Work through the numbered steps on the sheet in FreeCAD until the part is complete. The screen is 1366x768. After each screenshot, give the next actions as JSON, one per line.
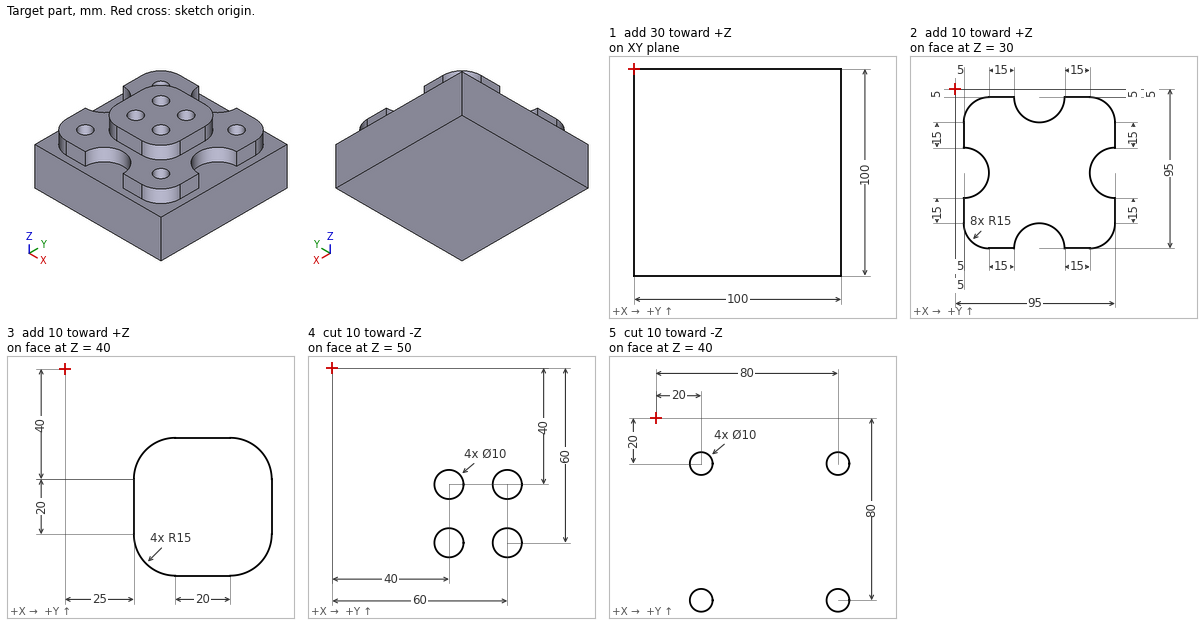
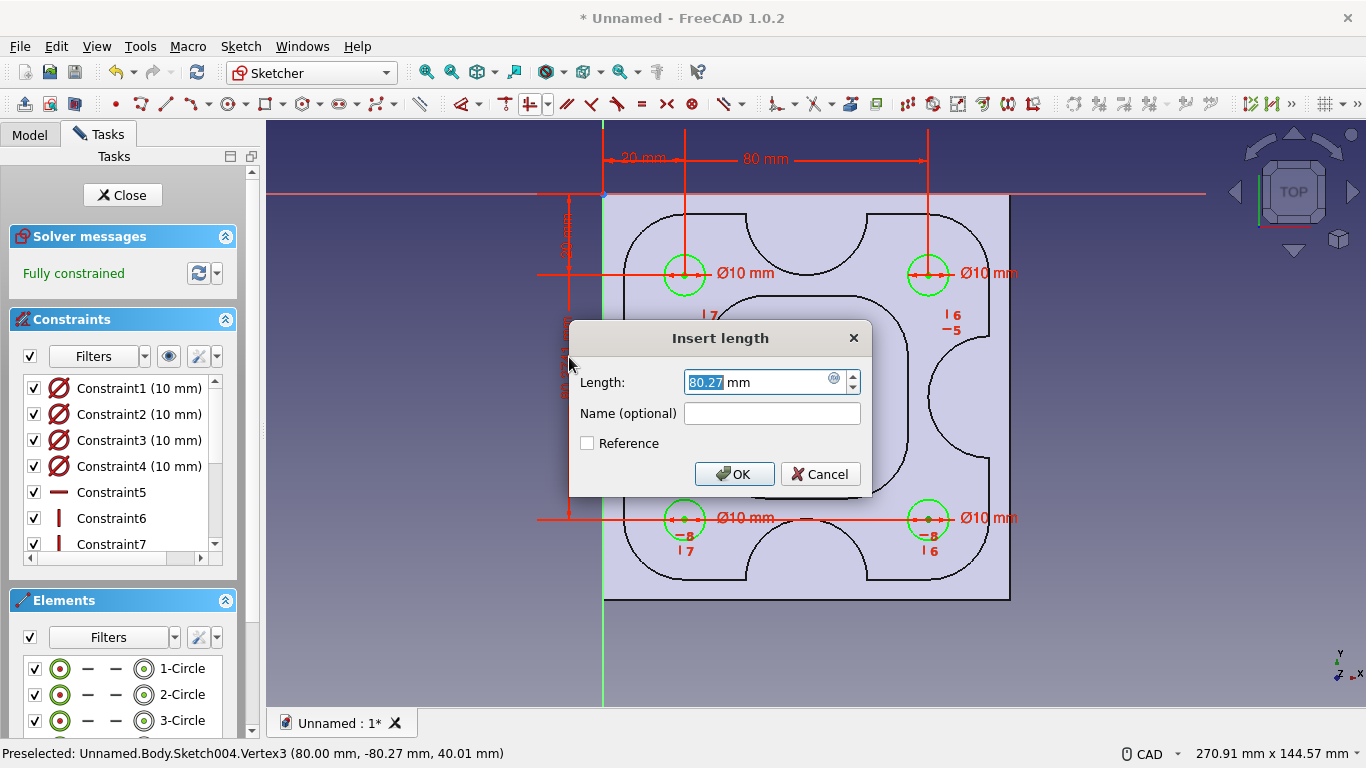
{"action": "type", "text": "80"}
{"action": "key", "text": "Return"}
{"action": "key", "text": "Escape"}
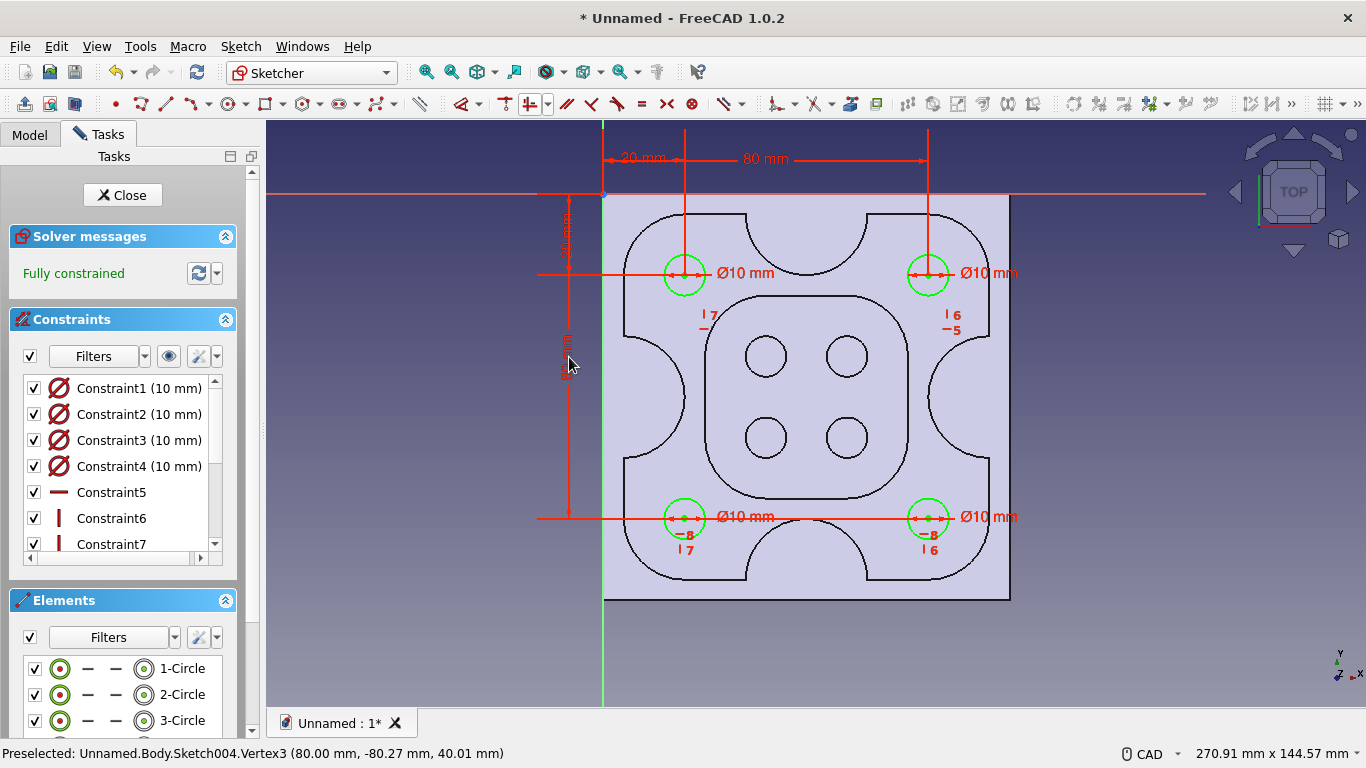
{"action": "left_click", "coordinate": [123, 195]}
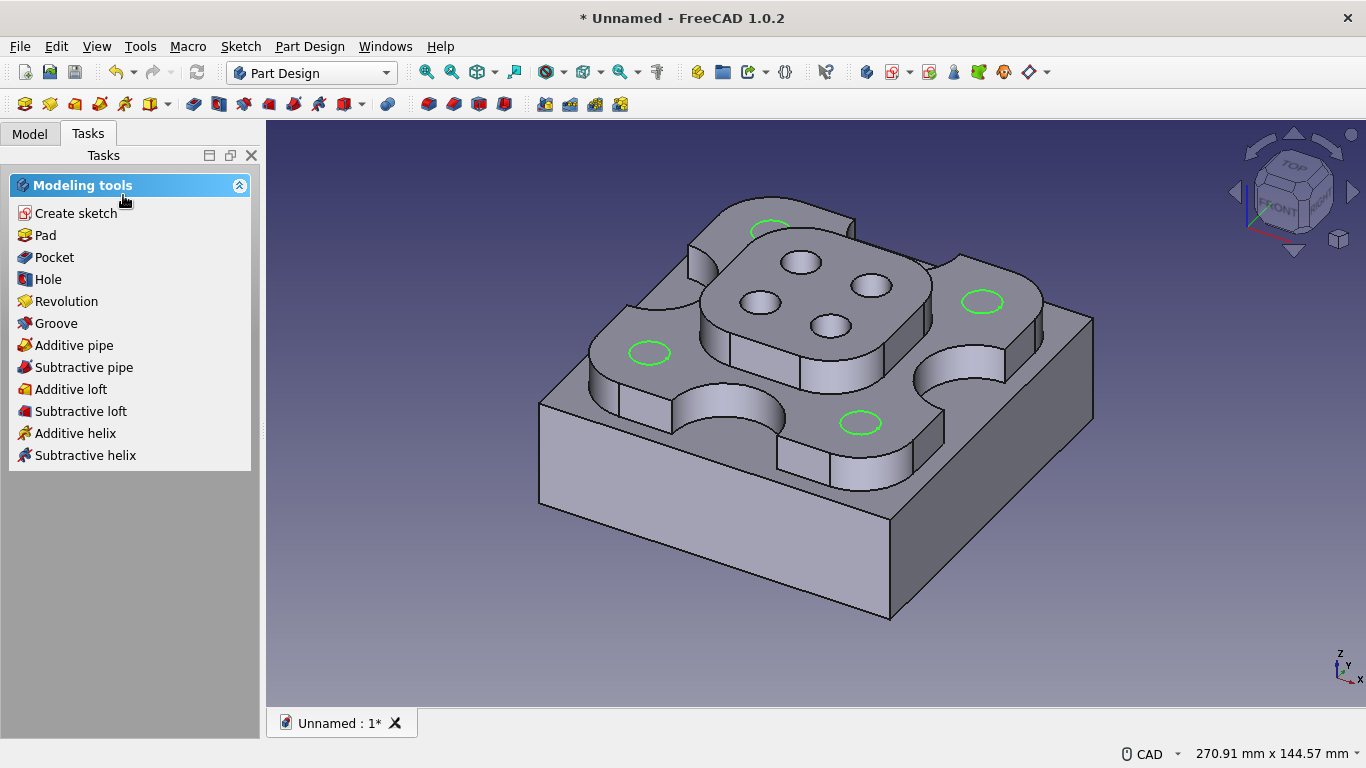
{"action": "left_click", "coordinate": [194, 104]}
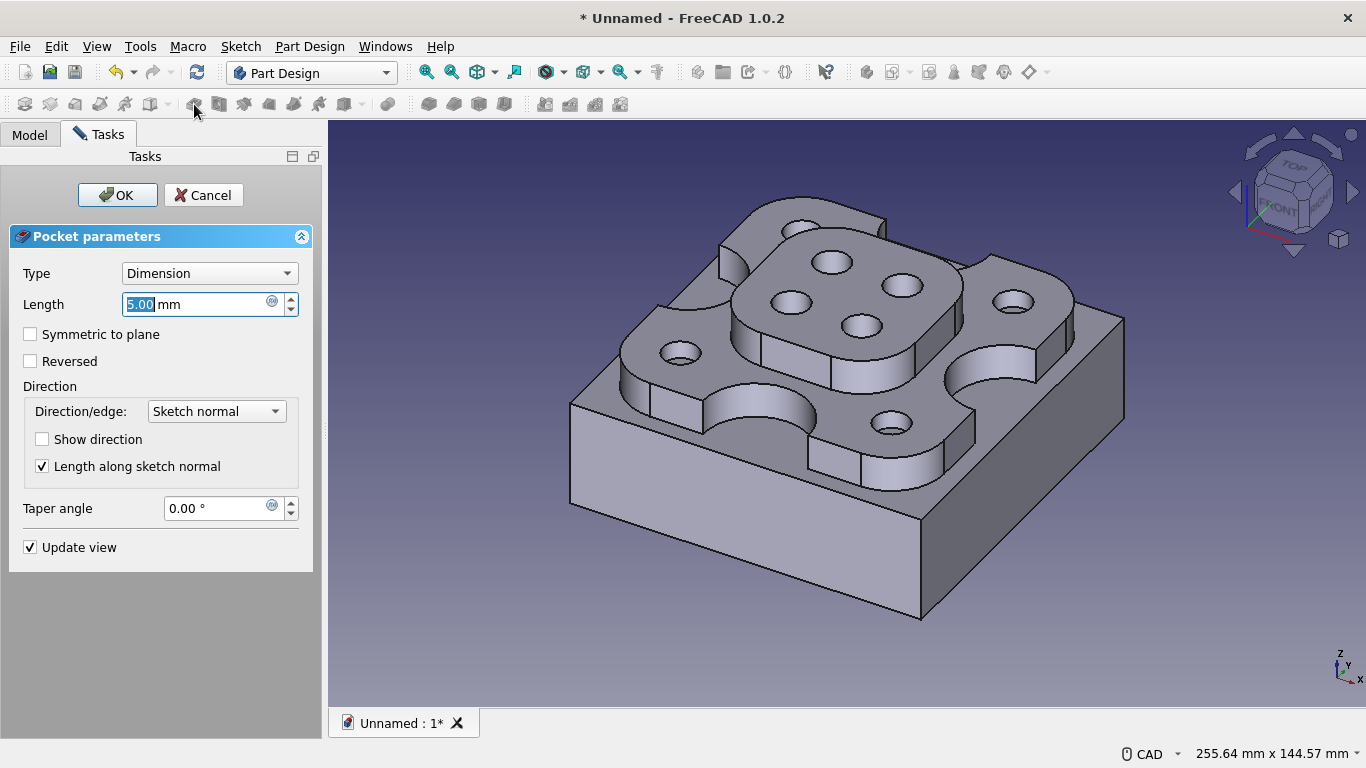
{"action": "type", "text": "10"}
{"action": "key", "text": "Tab"}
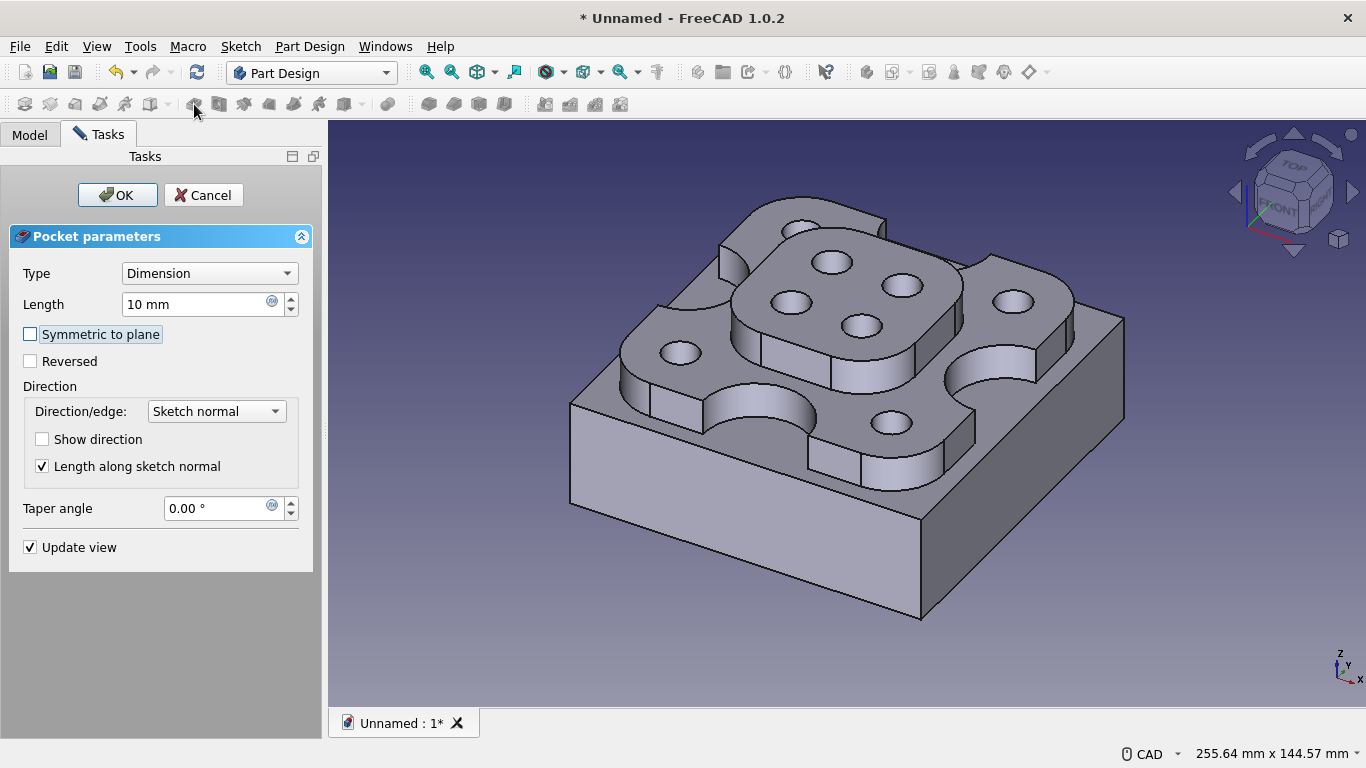
{"action": "left_click", "coordinate": [118, 195]}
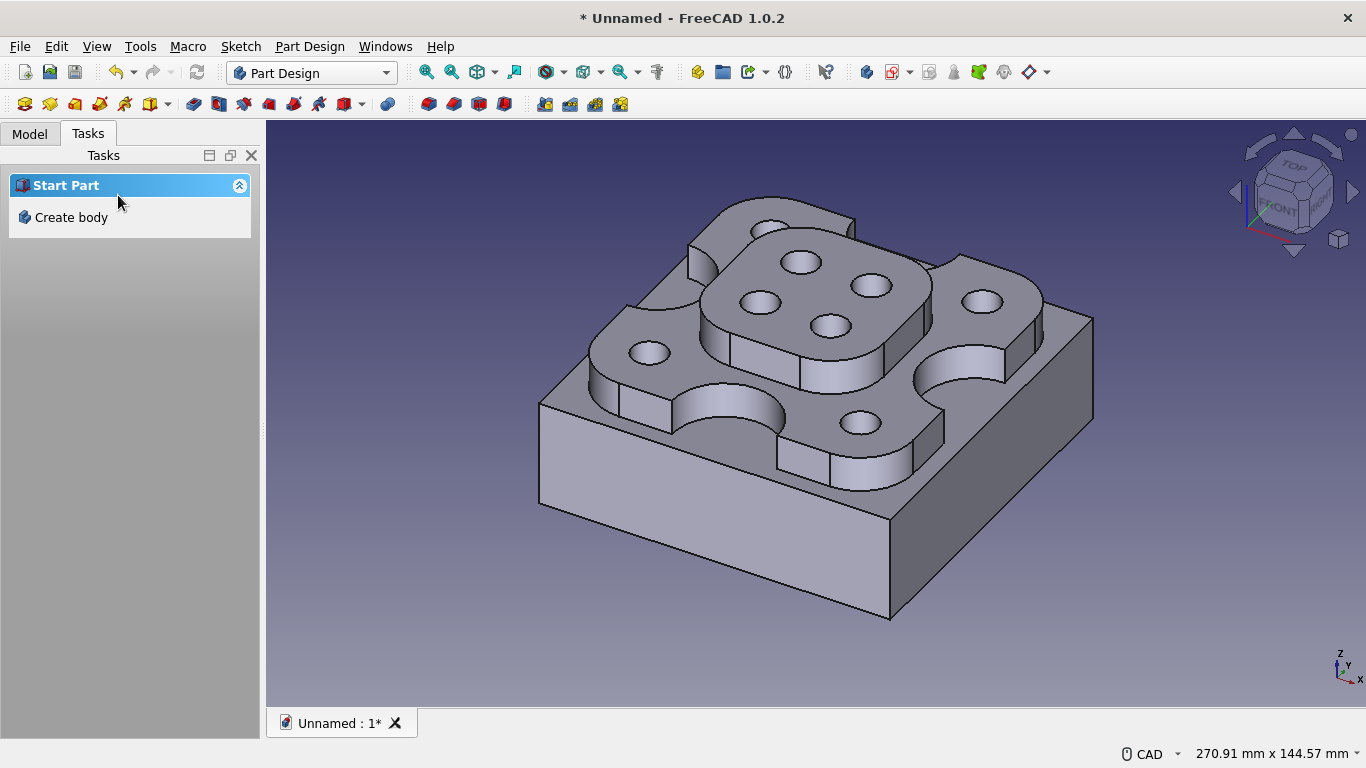
{"action": "key", "text": "0"}